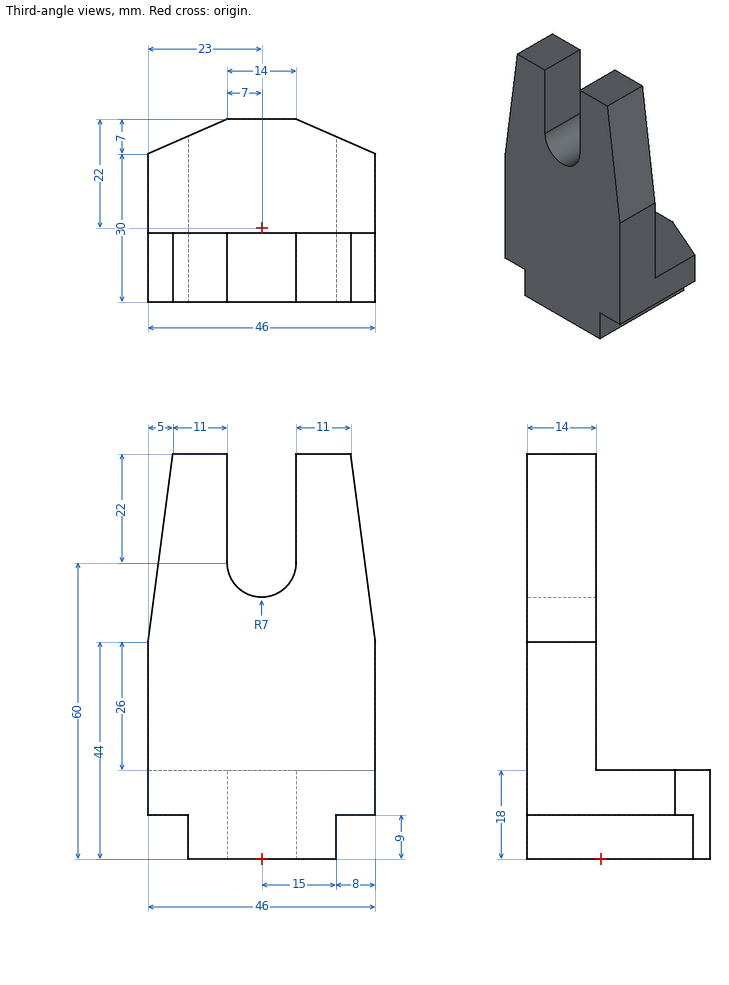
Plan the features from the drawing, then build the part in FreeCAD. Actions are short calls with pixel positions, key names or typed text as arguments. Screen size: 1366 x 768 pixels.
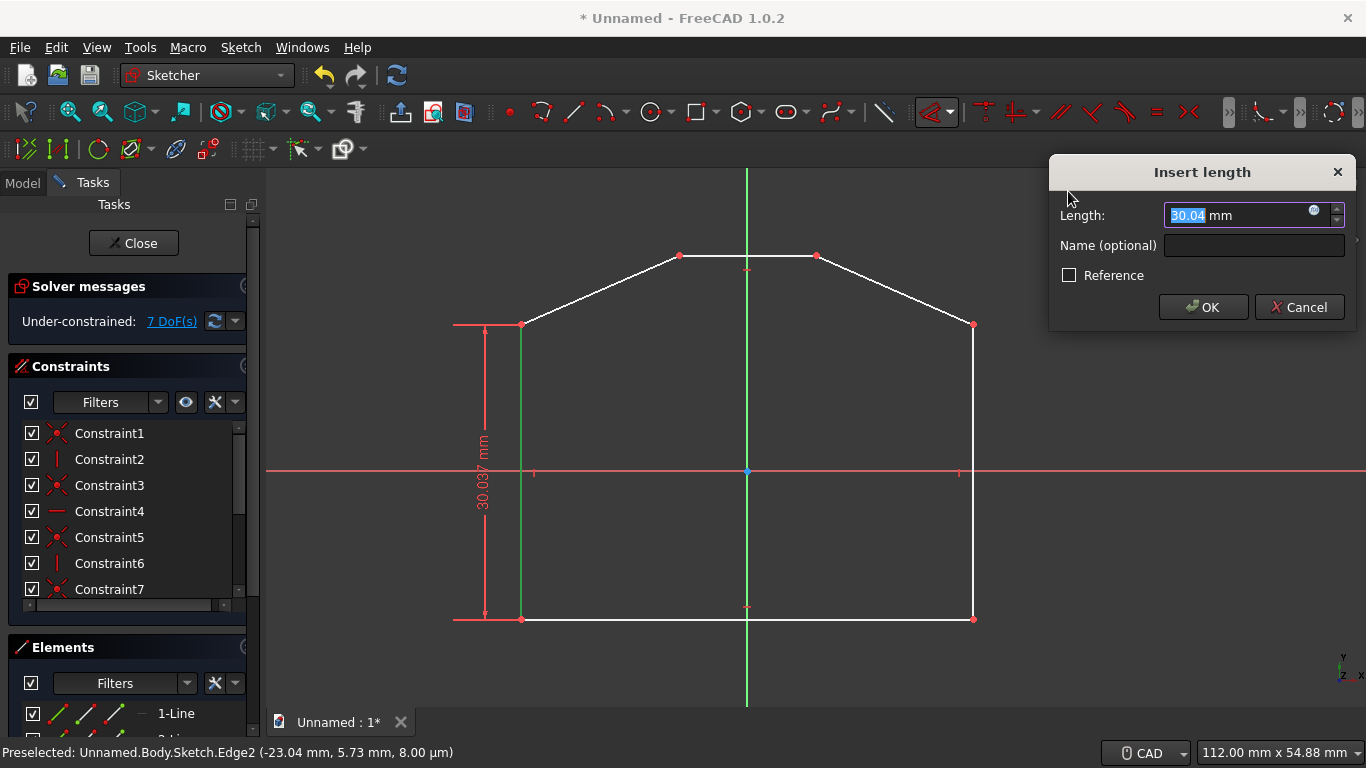
text(30)
key(Return)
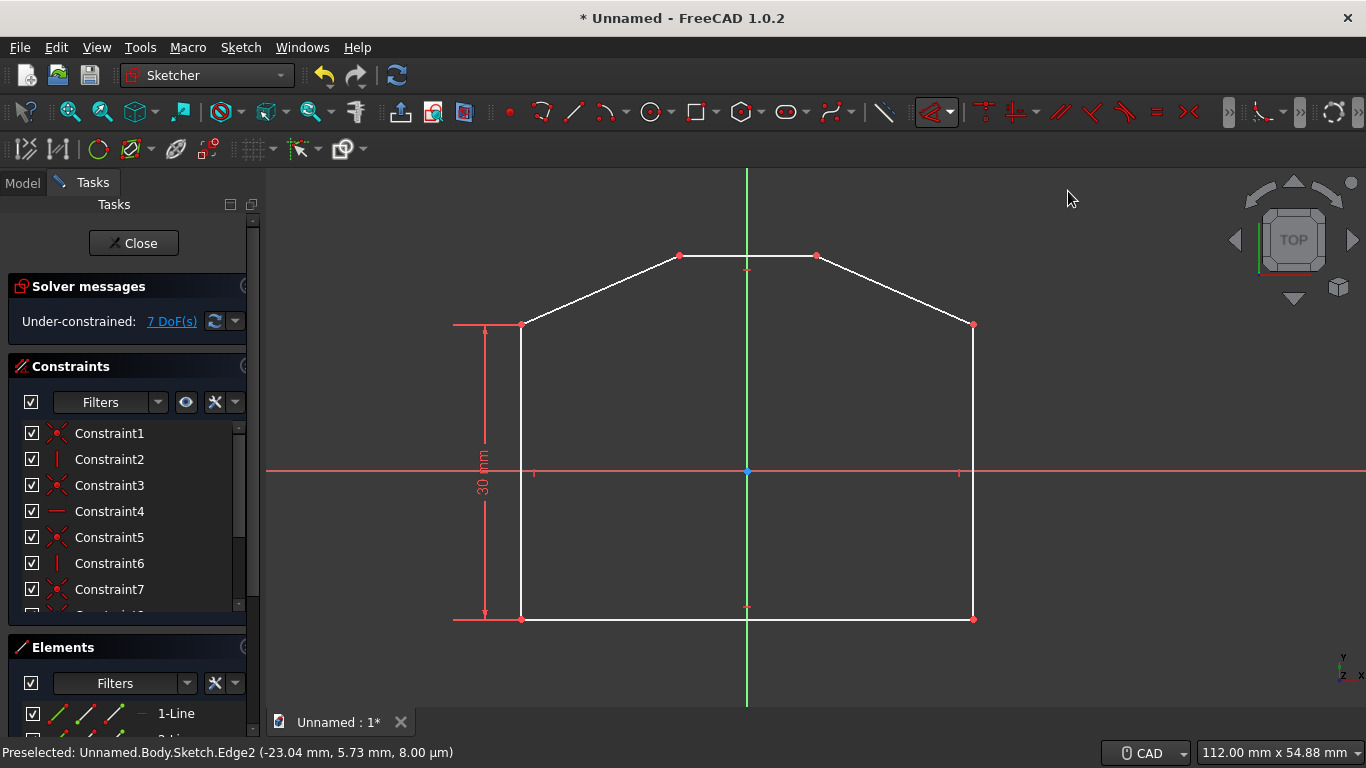
click(657, 620)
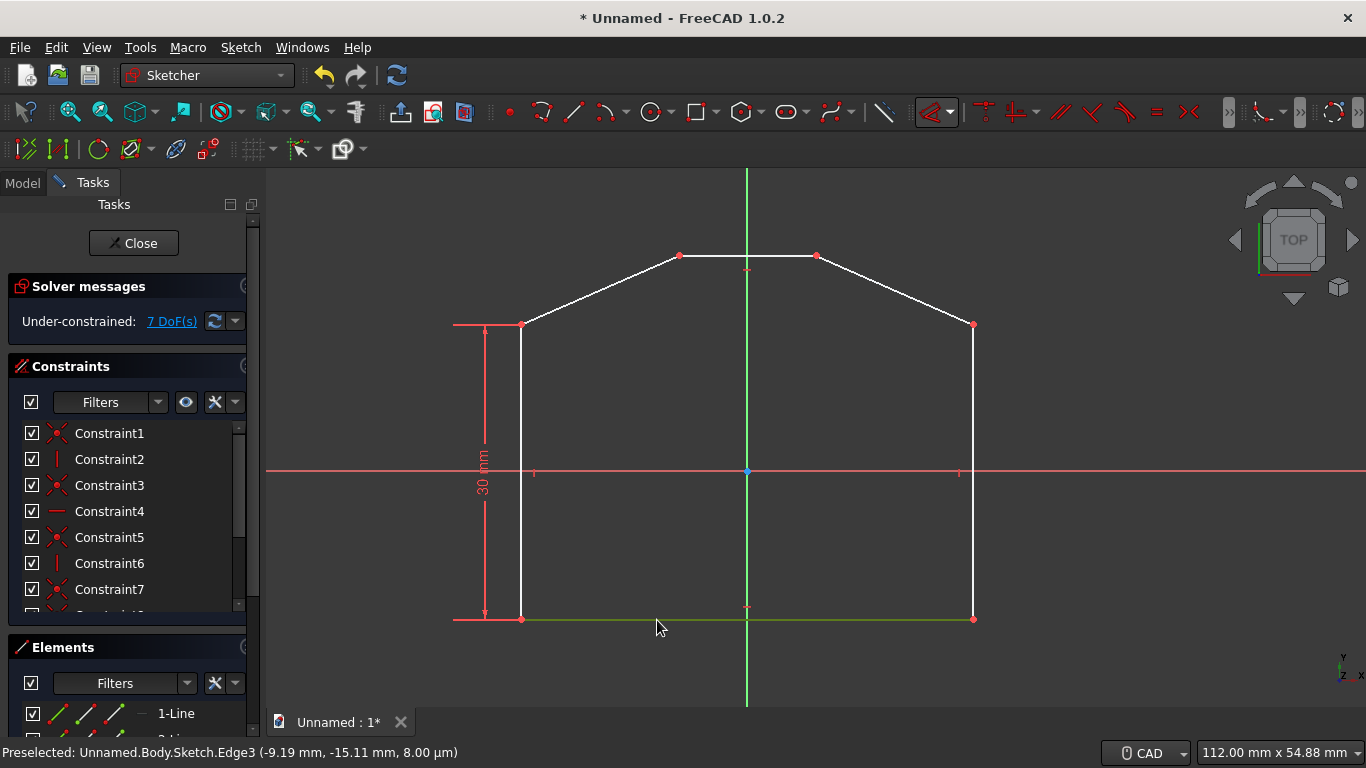
key(l)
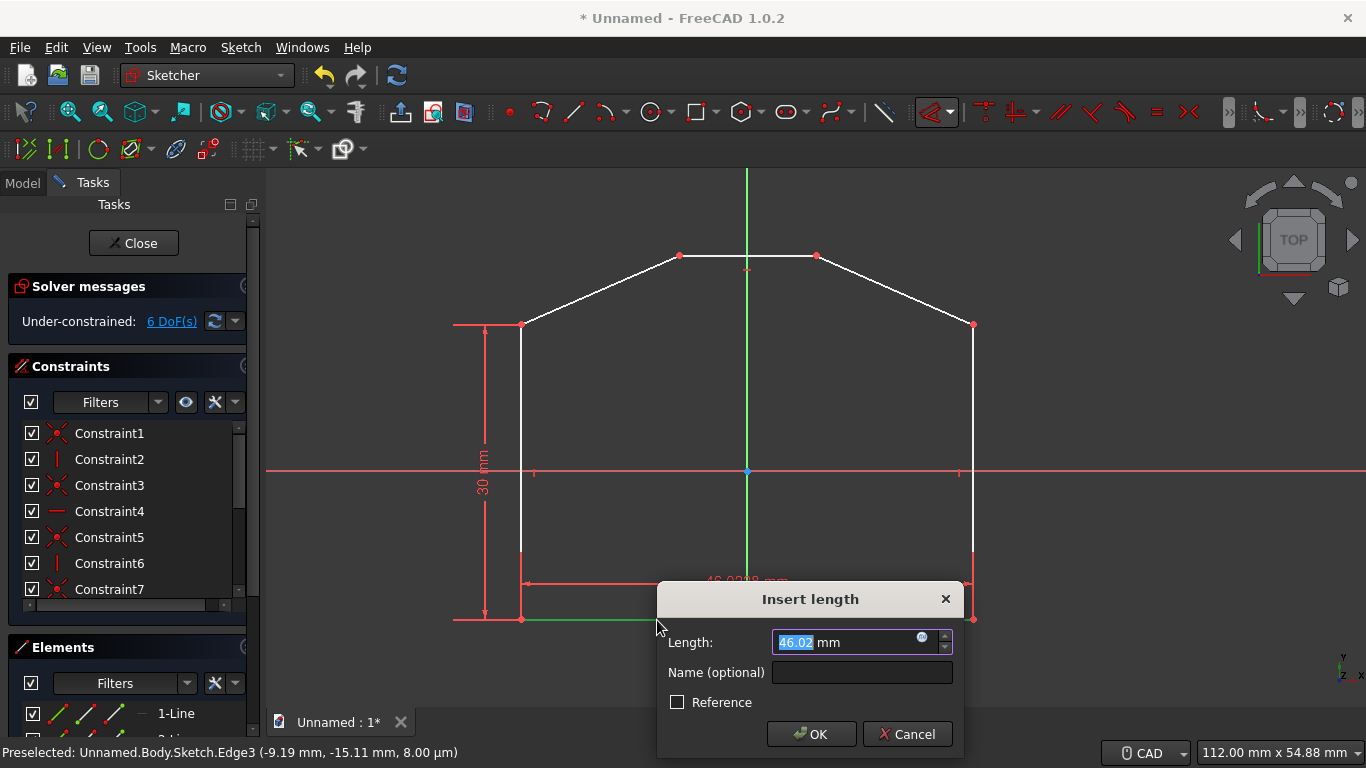
text(46)
key(Return)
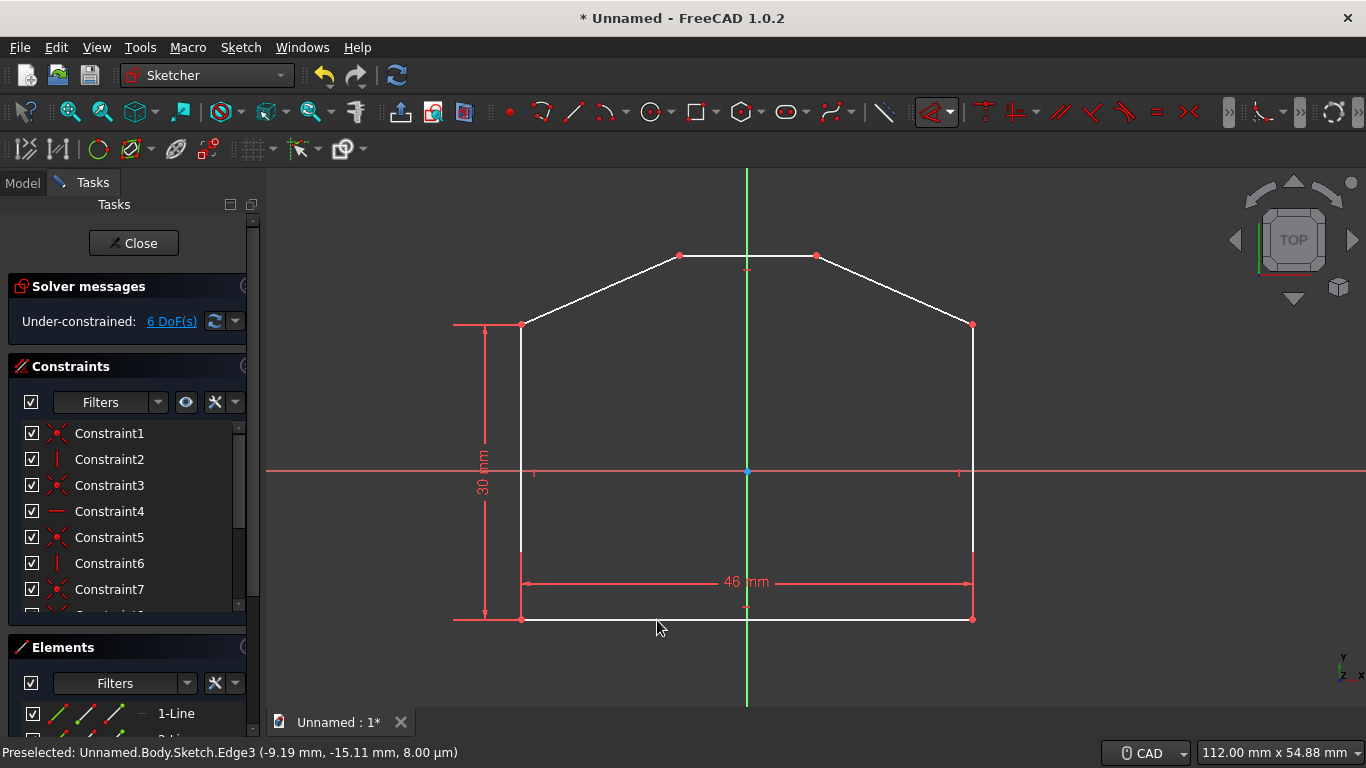
click(973, 531)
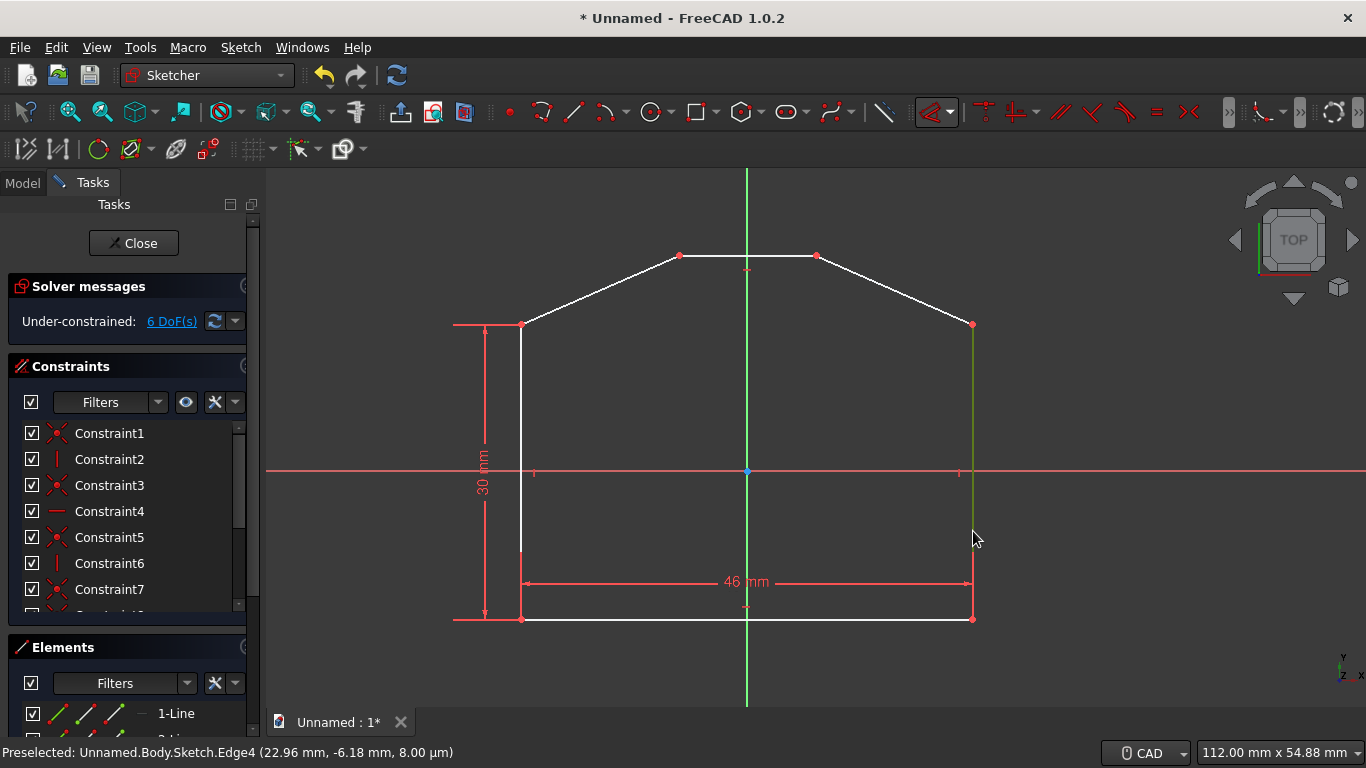
key(i)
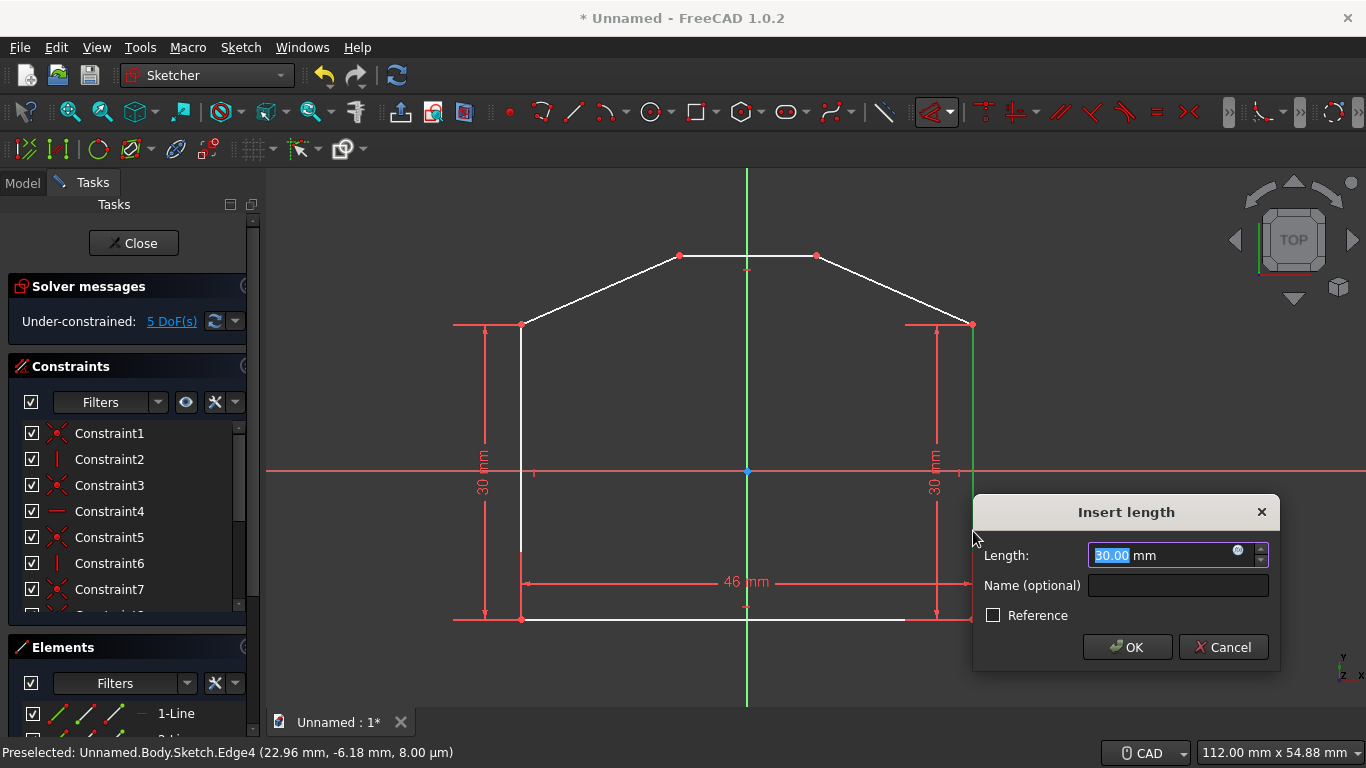
text(30)
key(Return)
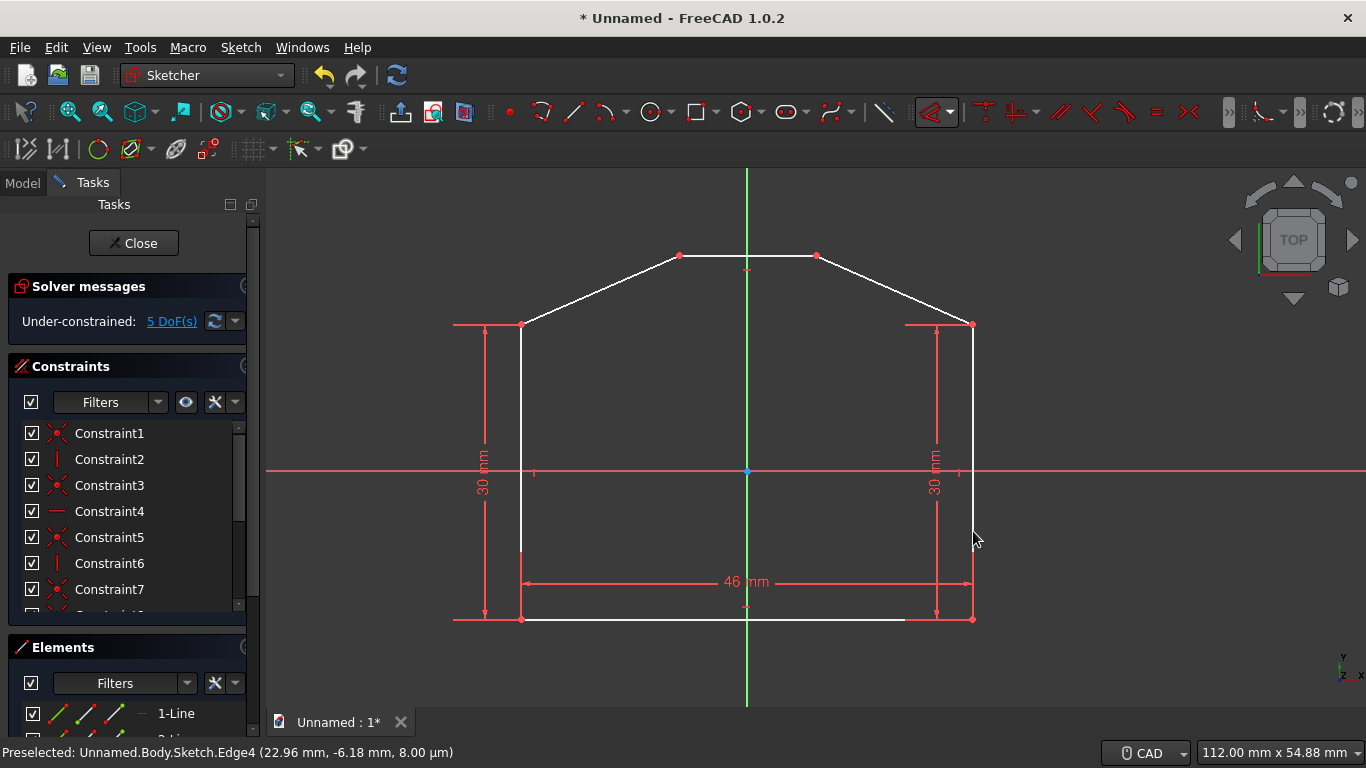
click(775, 256)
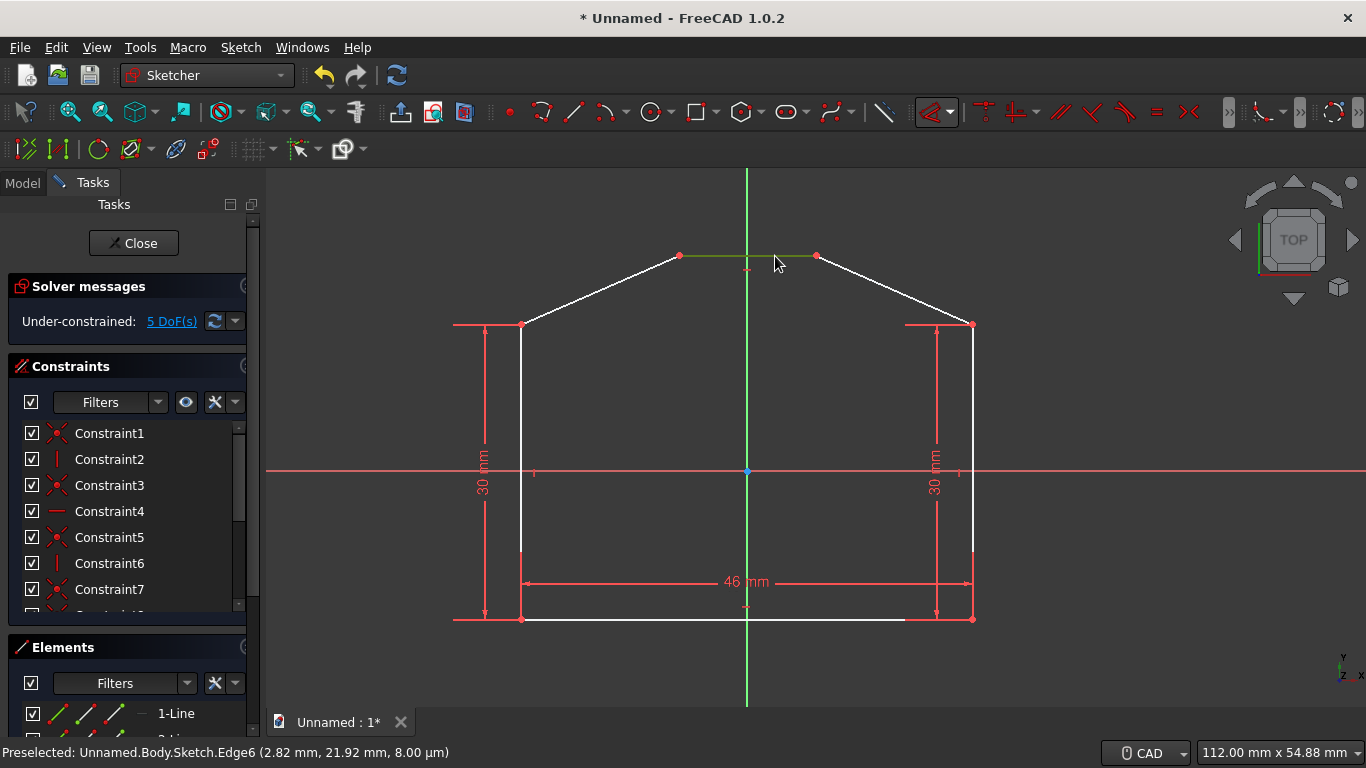
click(952, 112)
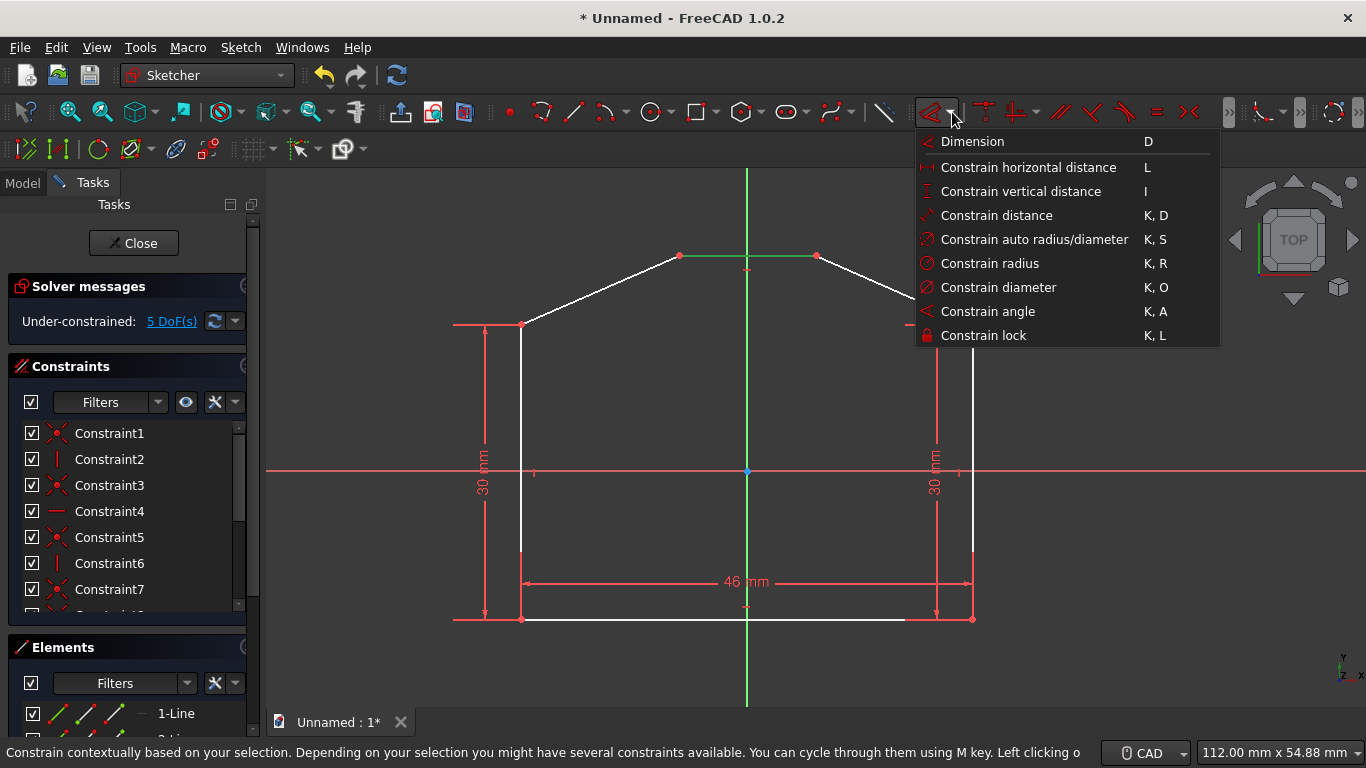
click(1068, 167)